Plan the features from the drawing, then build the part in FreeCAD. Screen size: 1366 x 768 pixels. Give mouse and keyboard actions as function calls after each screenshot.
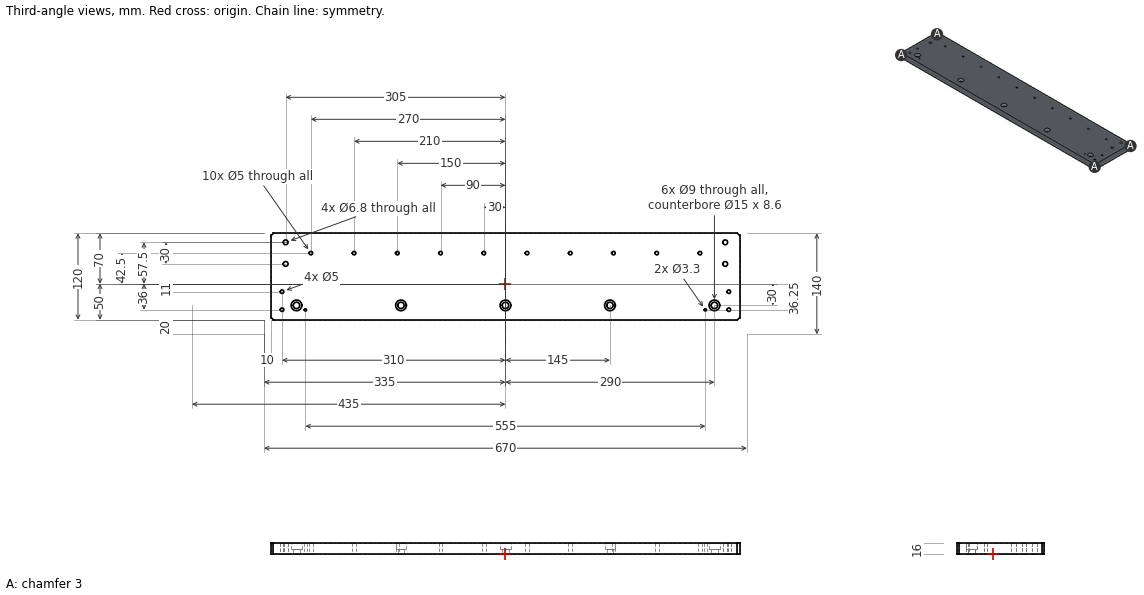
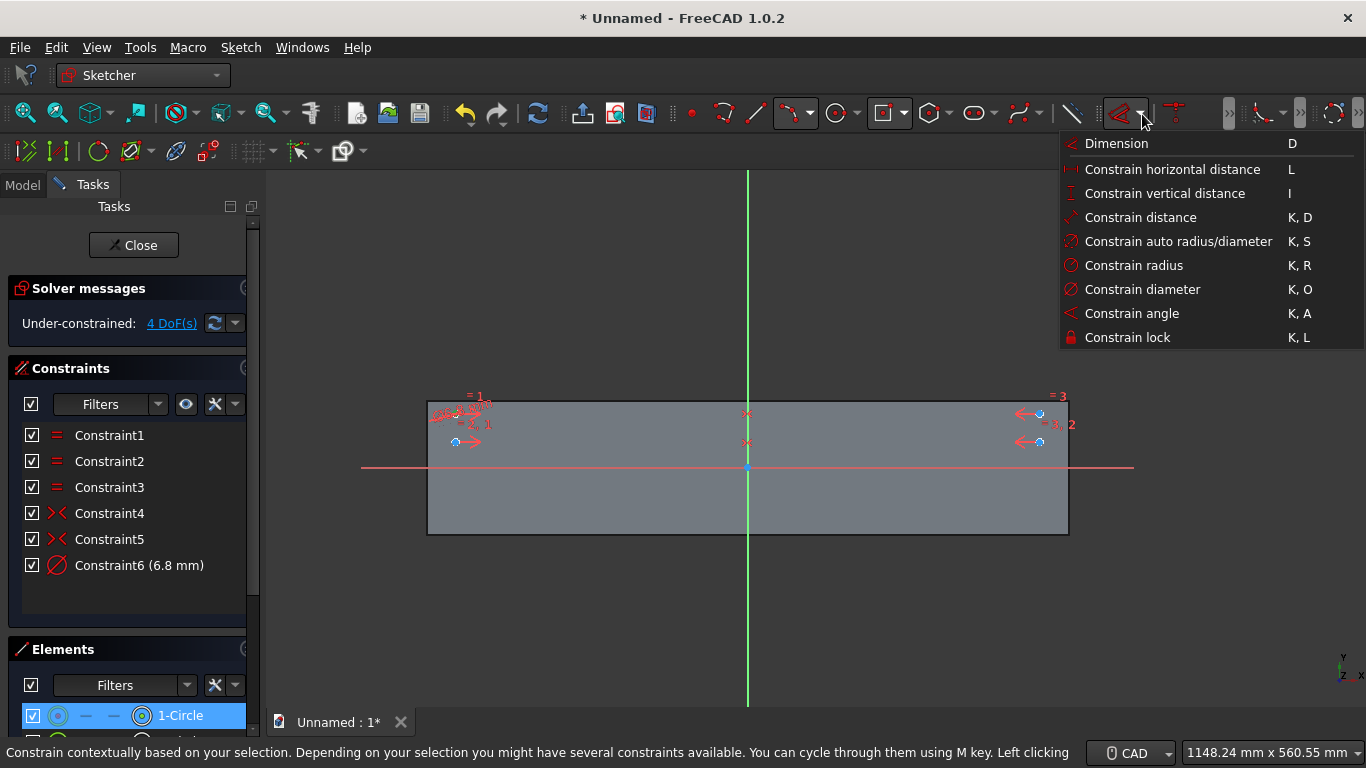
click(1212, 169)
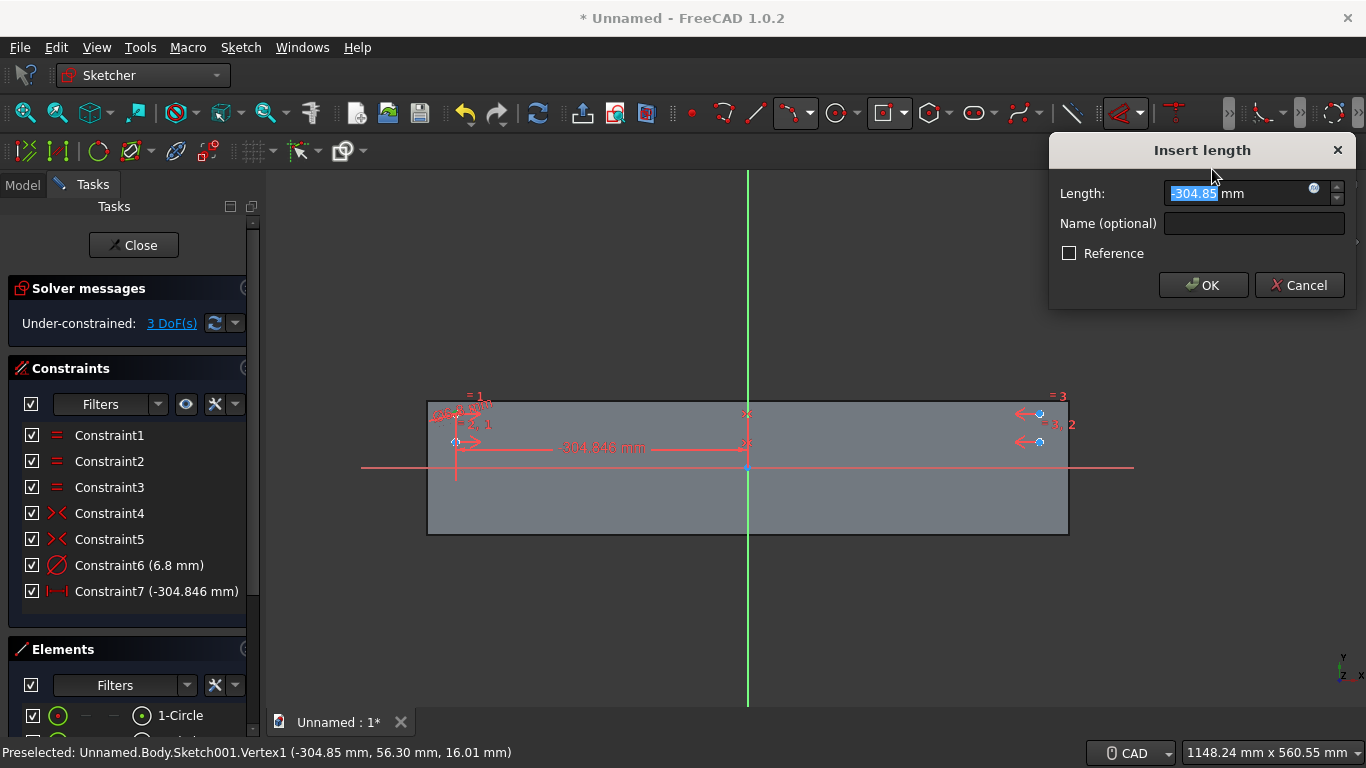
text(-305)
key(Return)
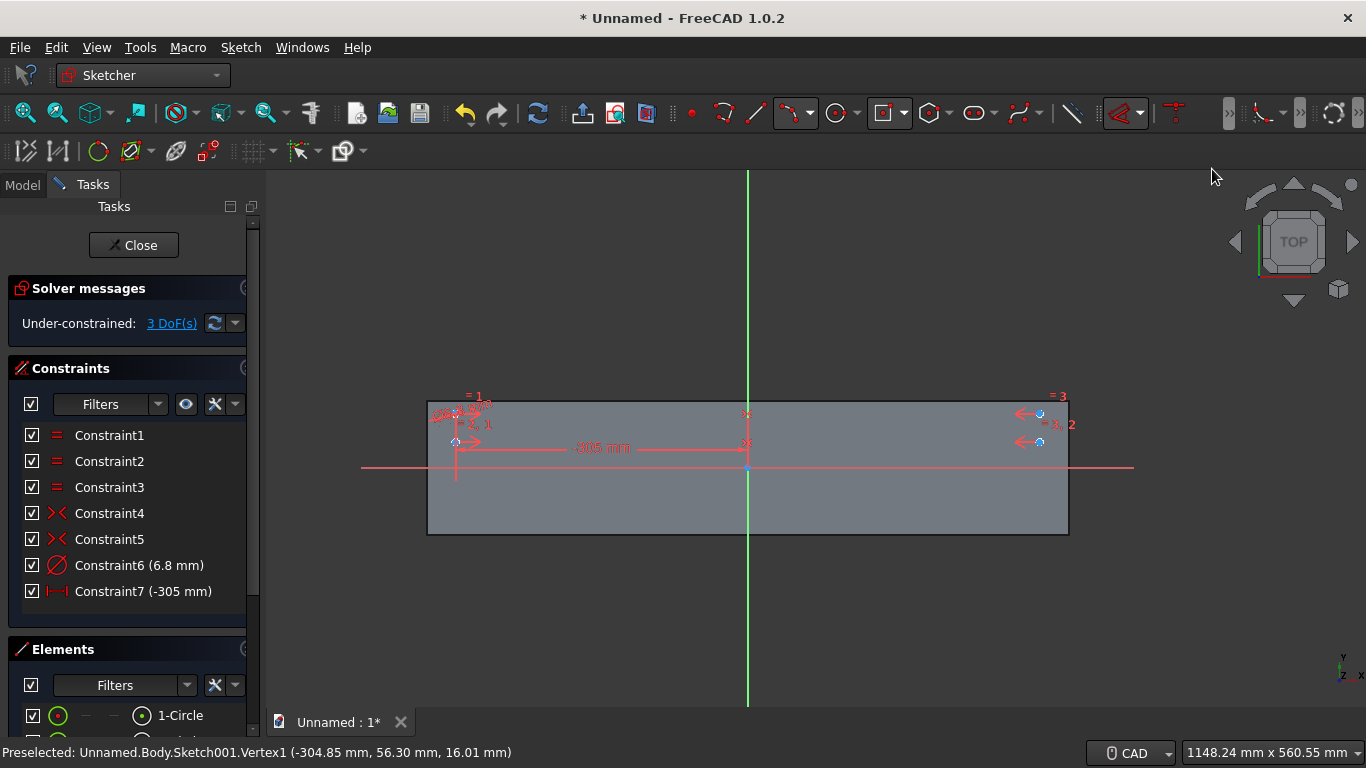
click(456, 442)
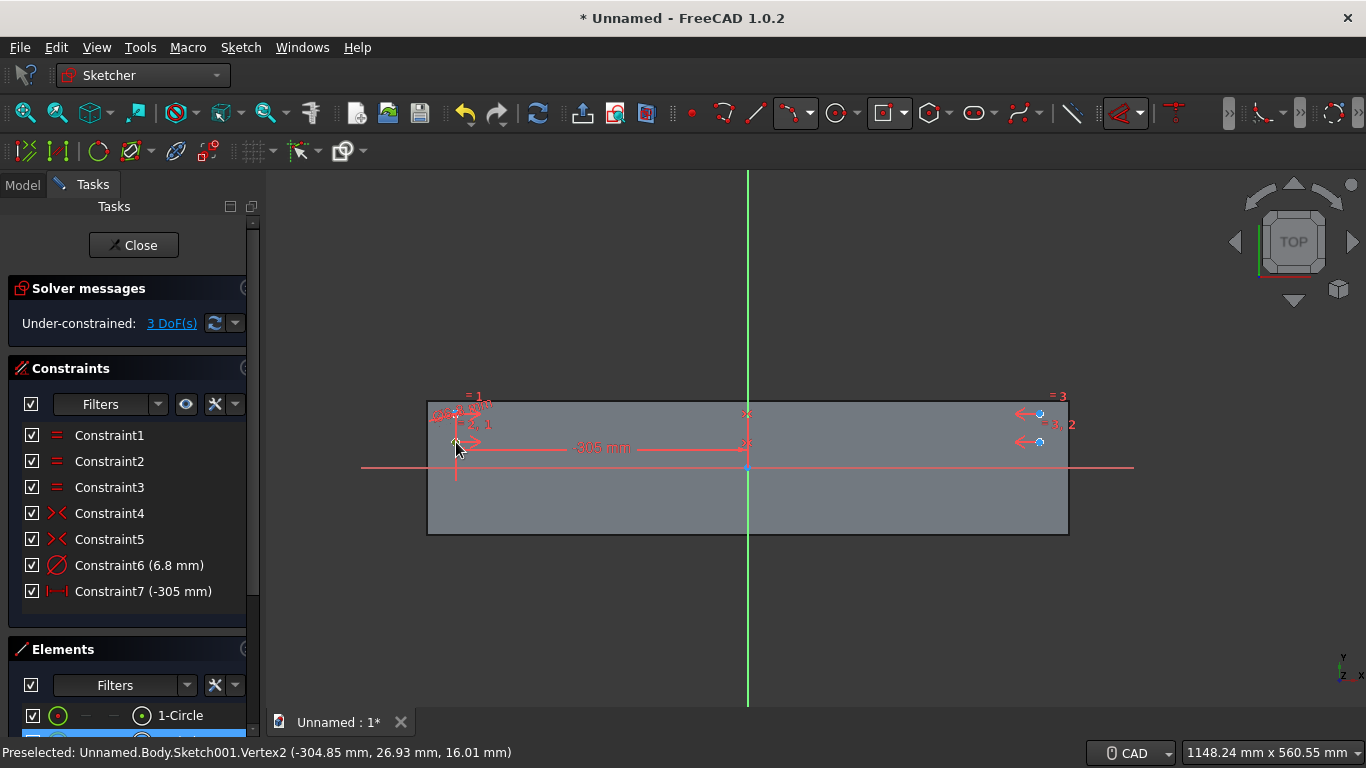
key(l)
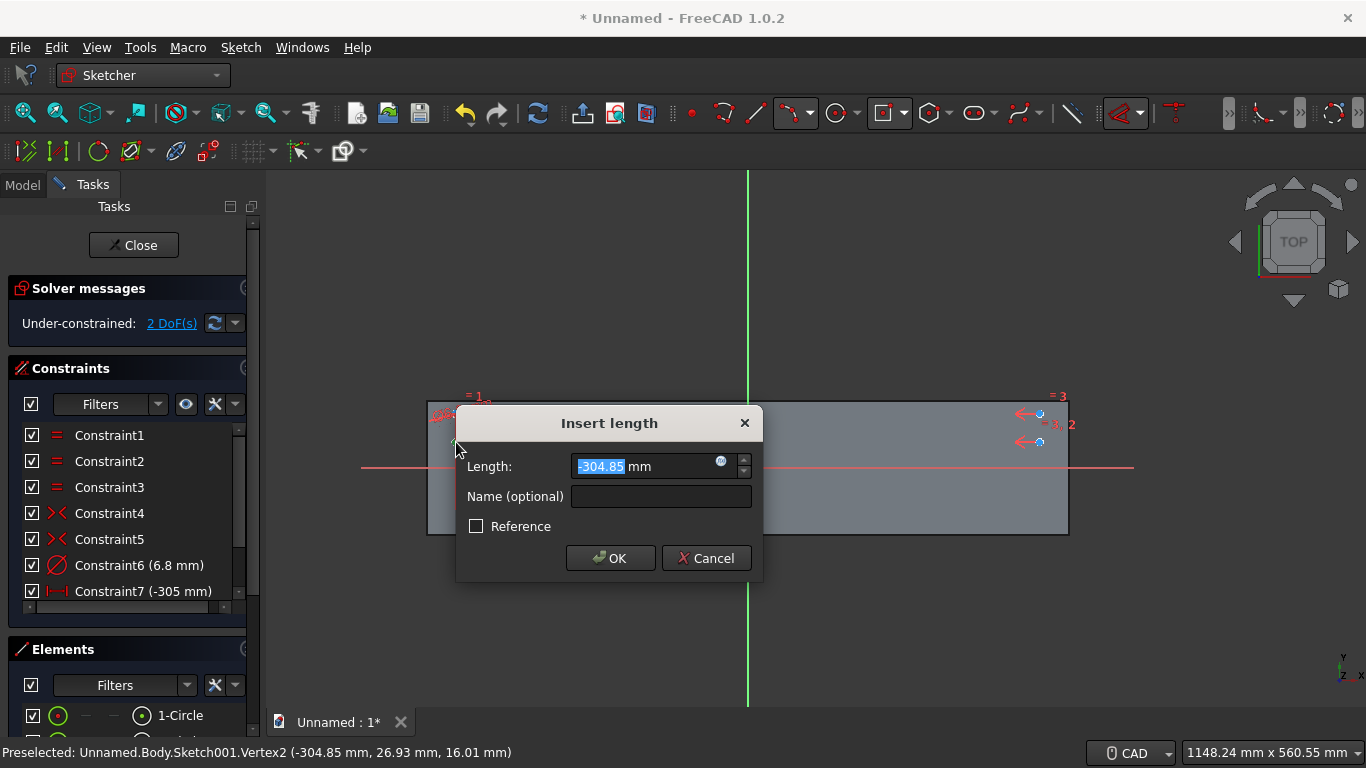
text(-305)
key(Return)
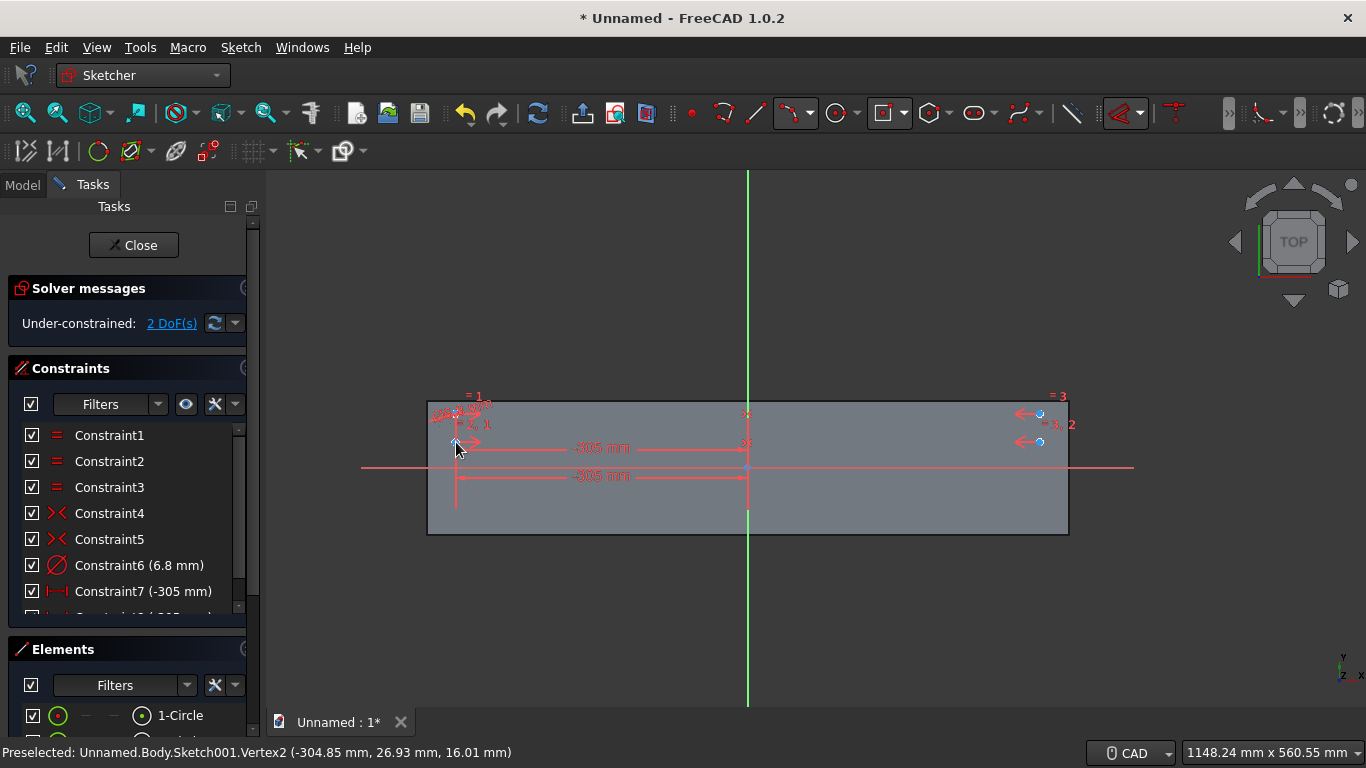
scroll(456, 414, up, 2)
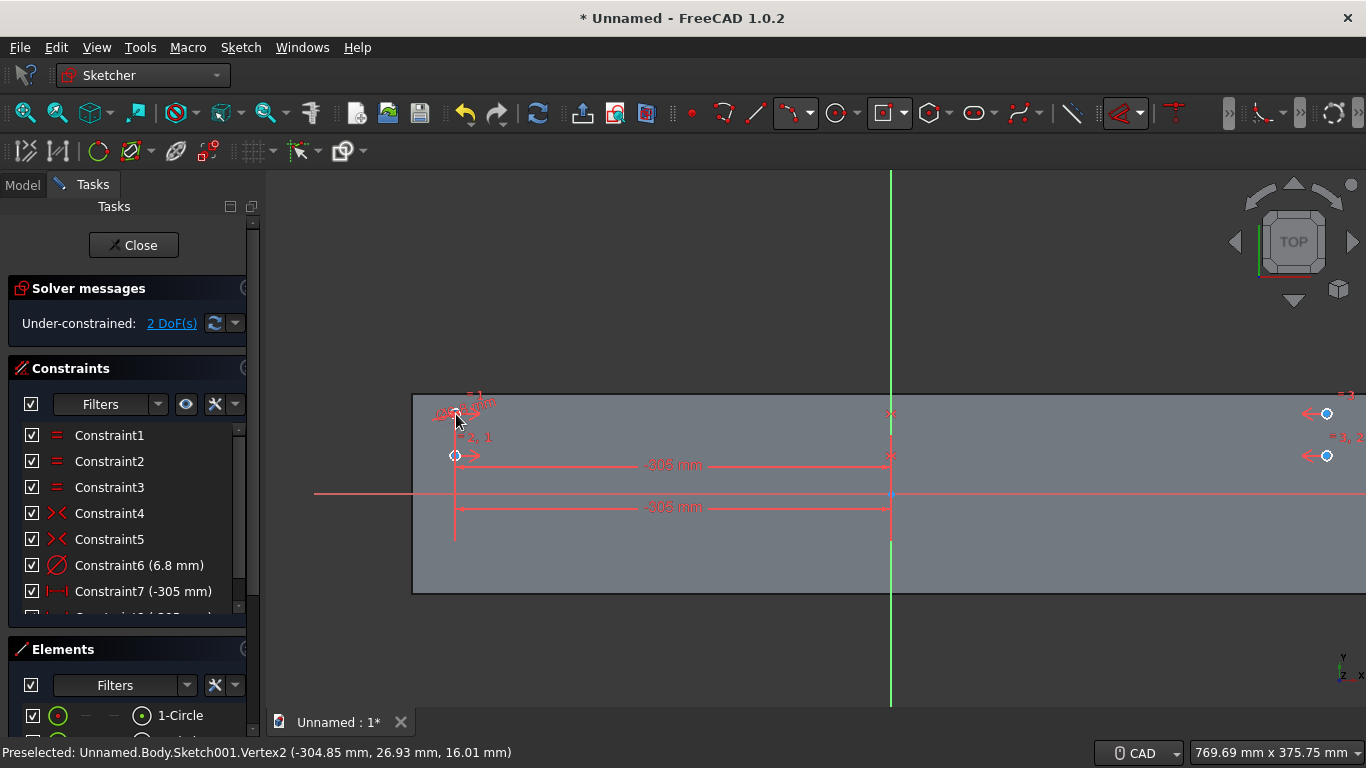
click(455, 414)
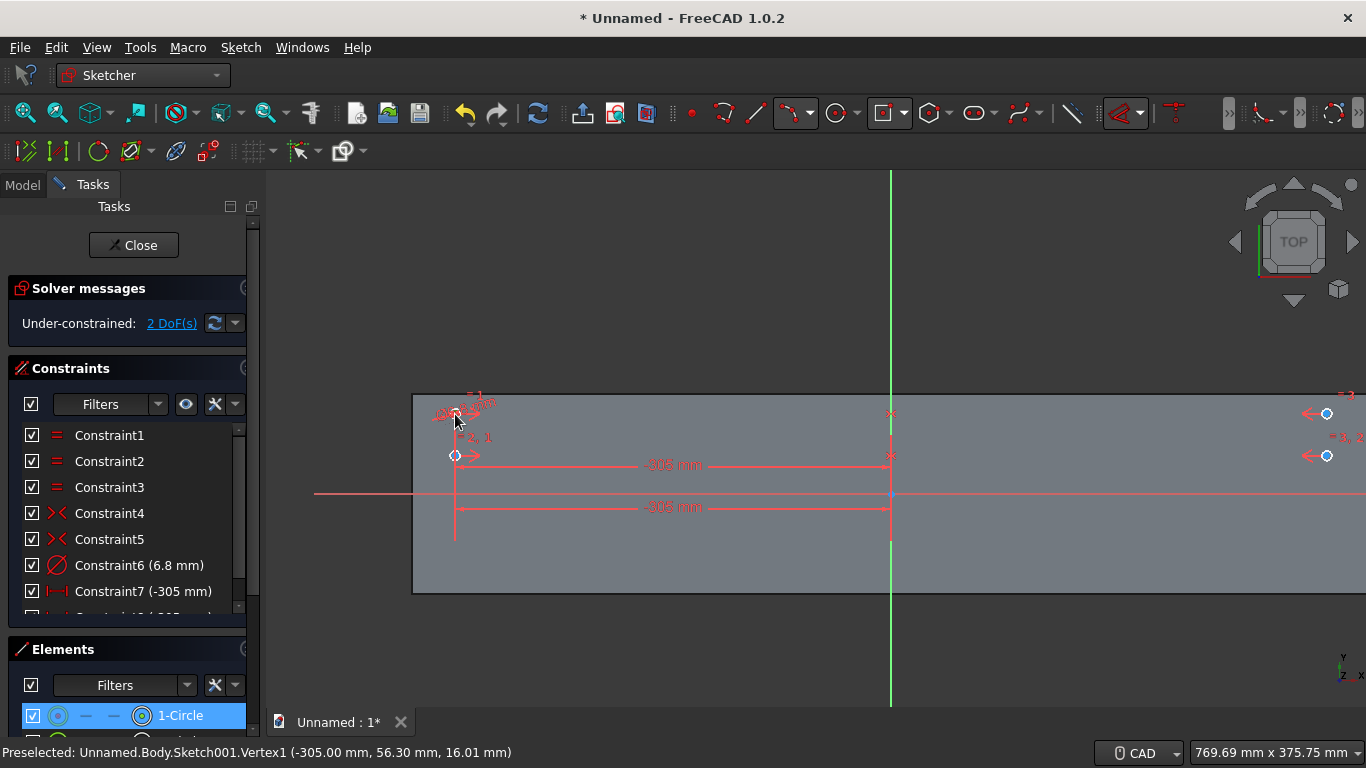
click(455, 456)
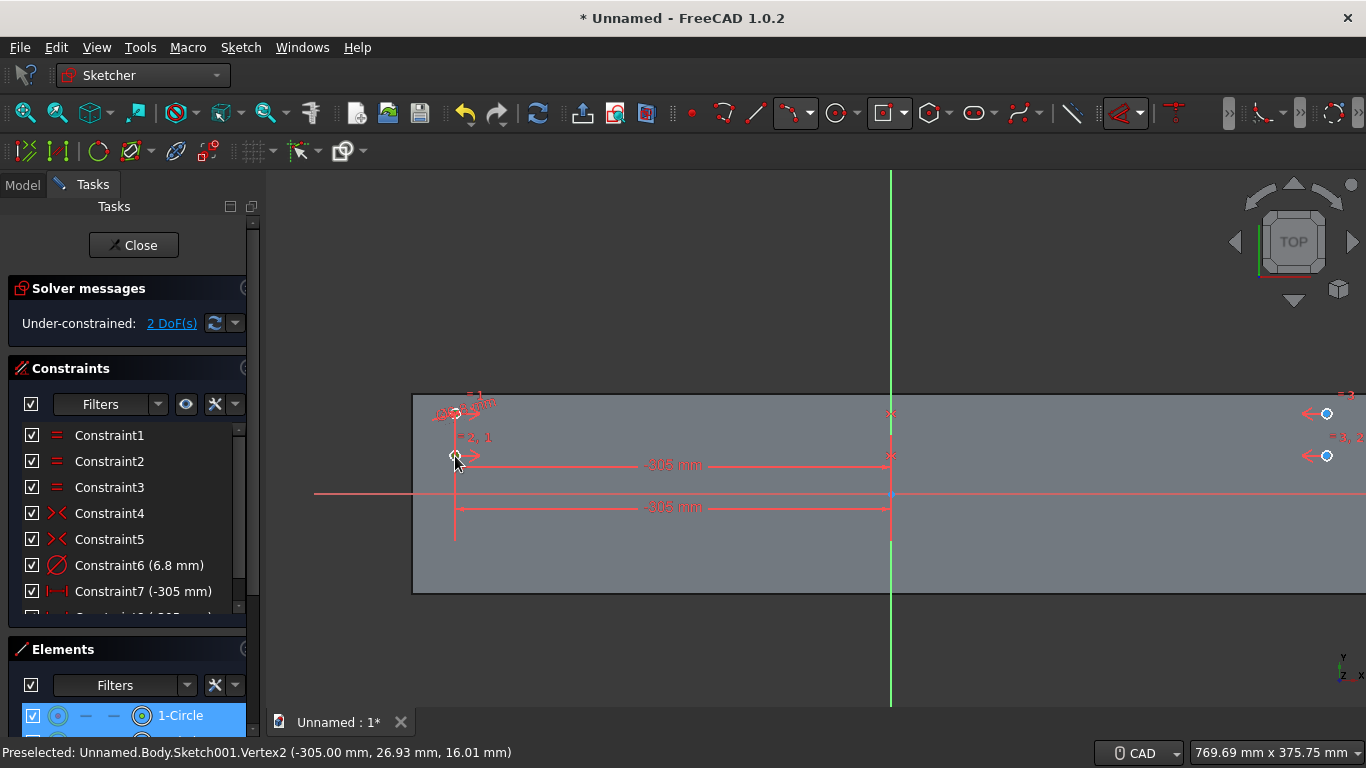
key(i)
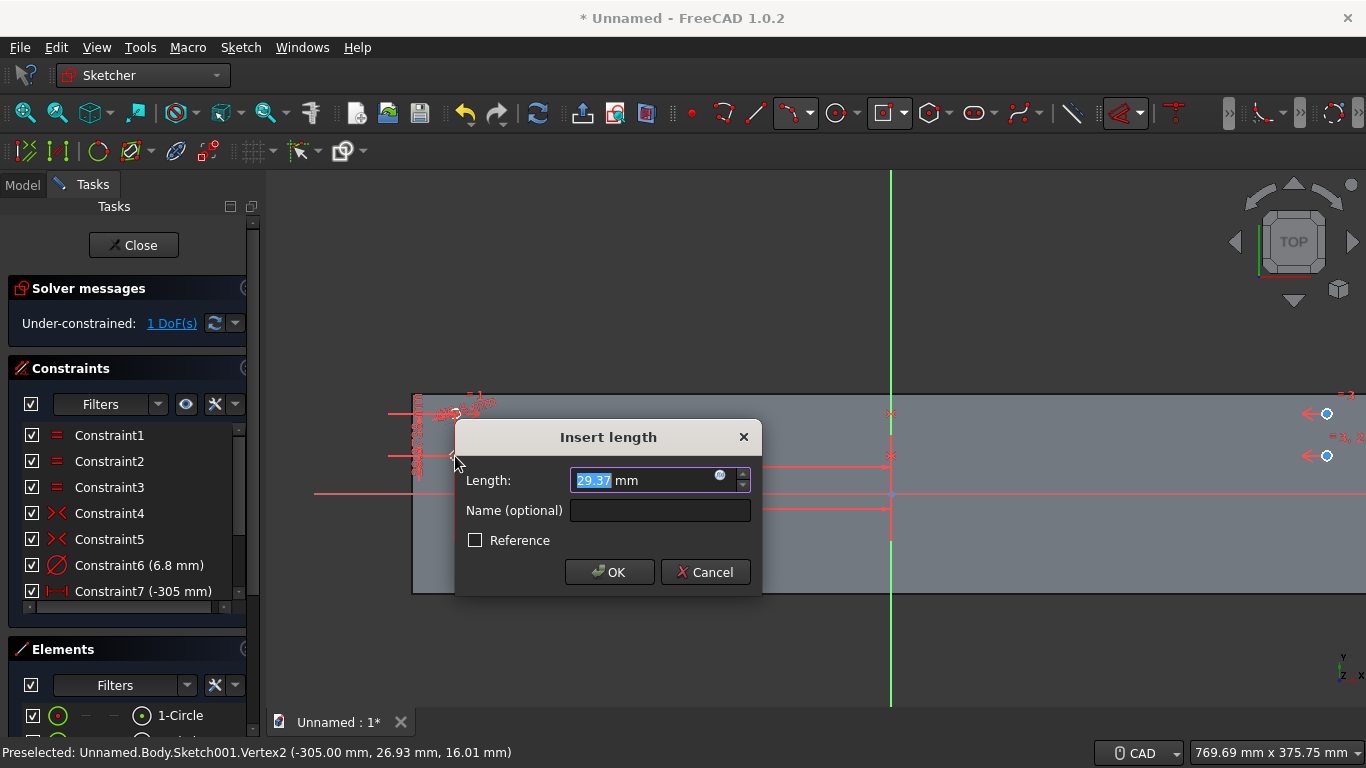
text(30)
key(Return)